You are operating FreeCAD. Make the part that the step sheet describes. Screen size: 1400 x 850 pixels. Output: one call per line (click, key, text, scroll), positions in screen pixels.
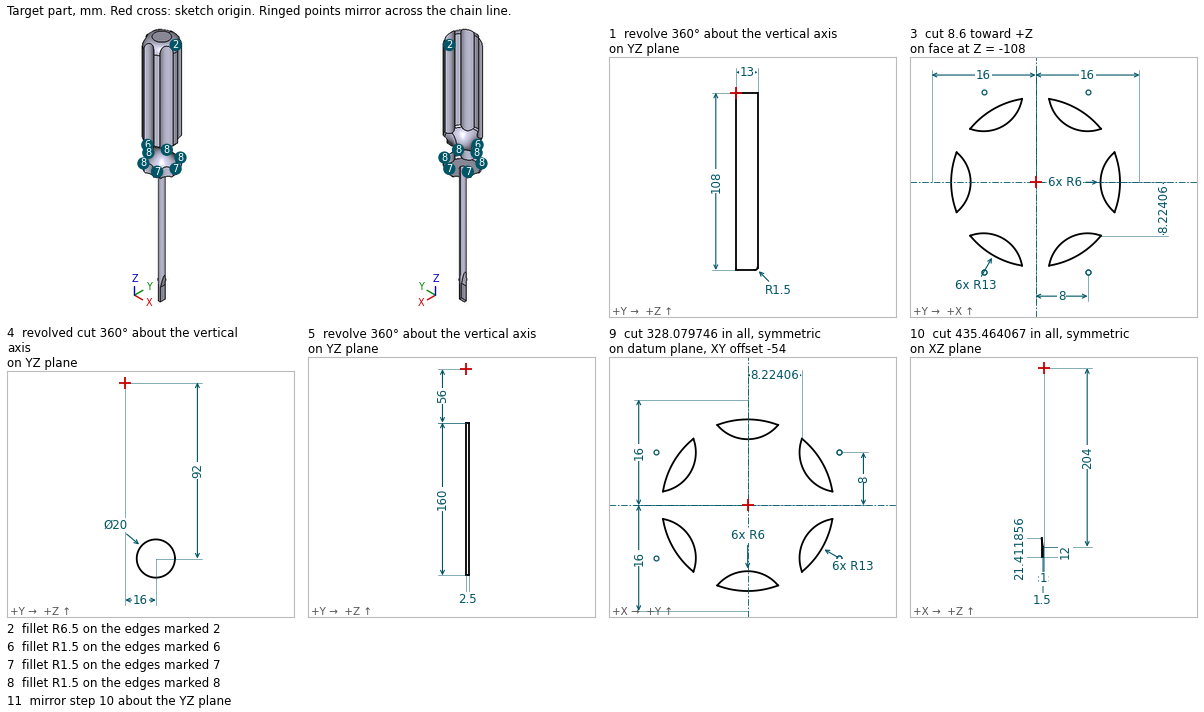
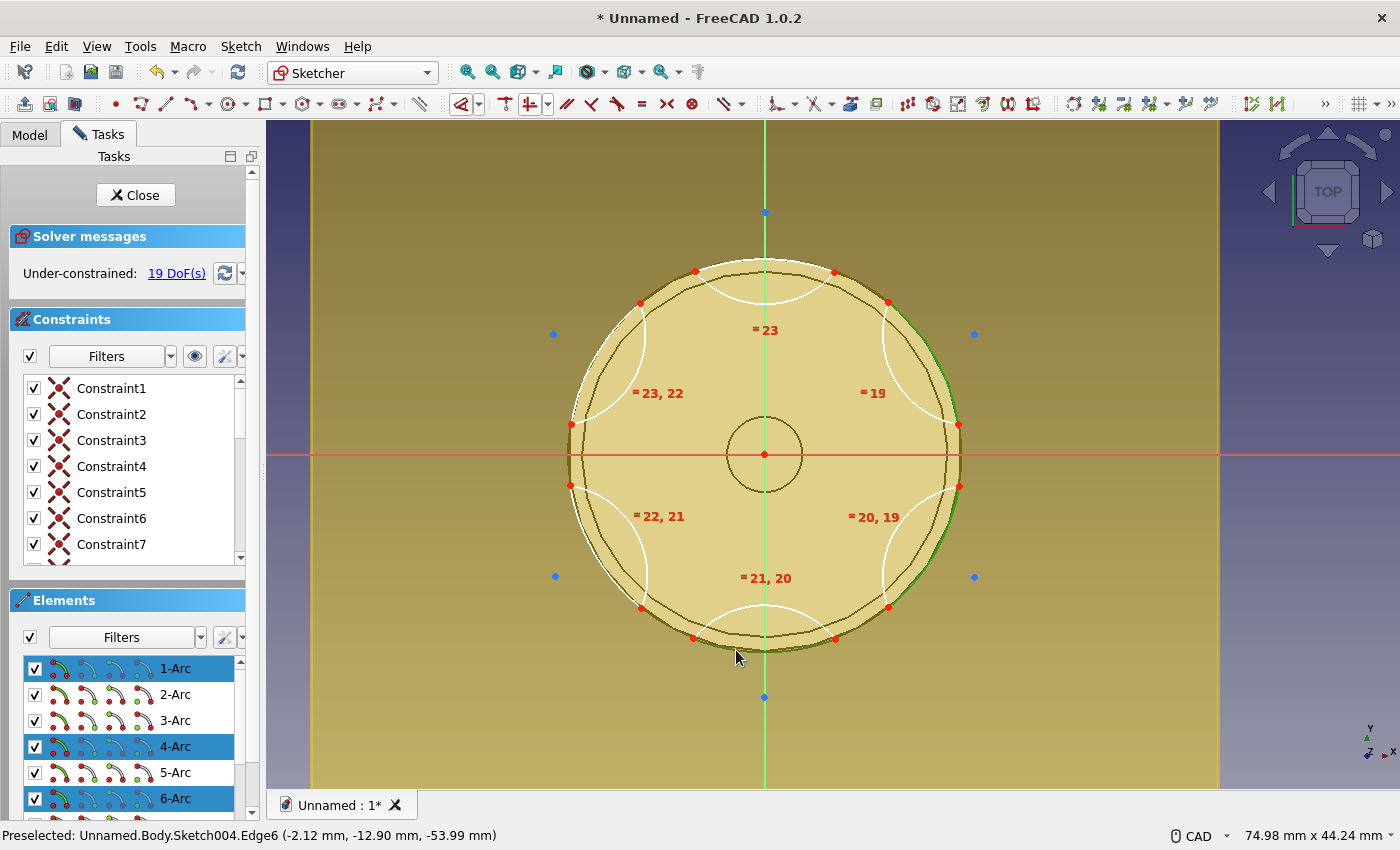
click(582, 528)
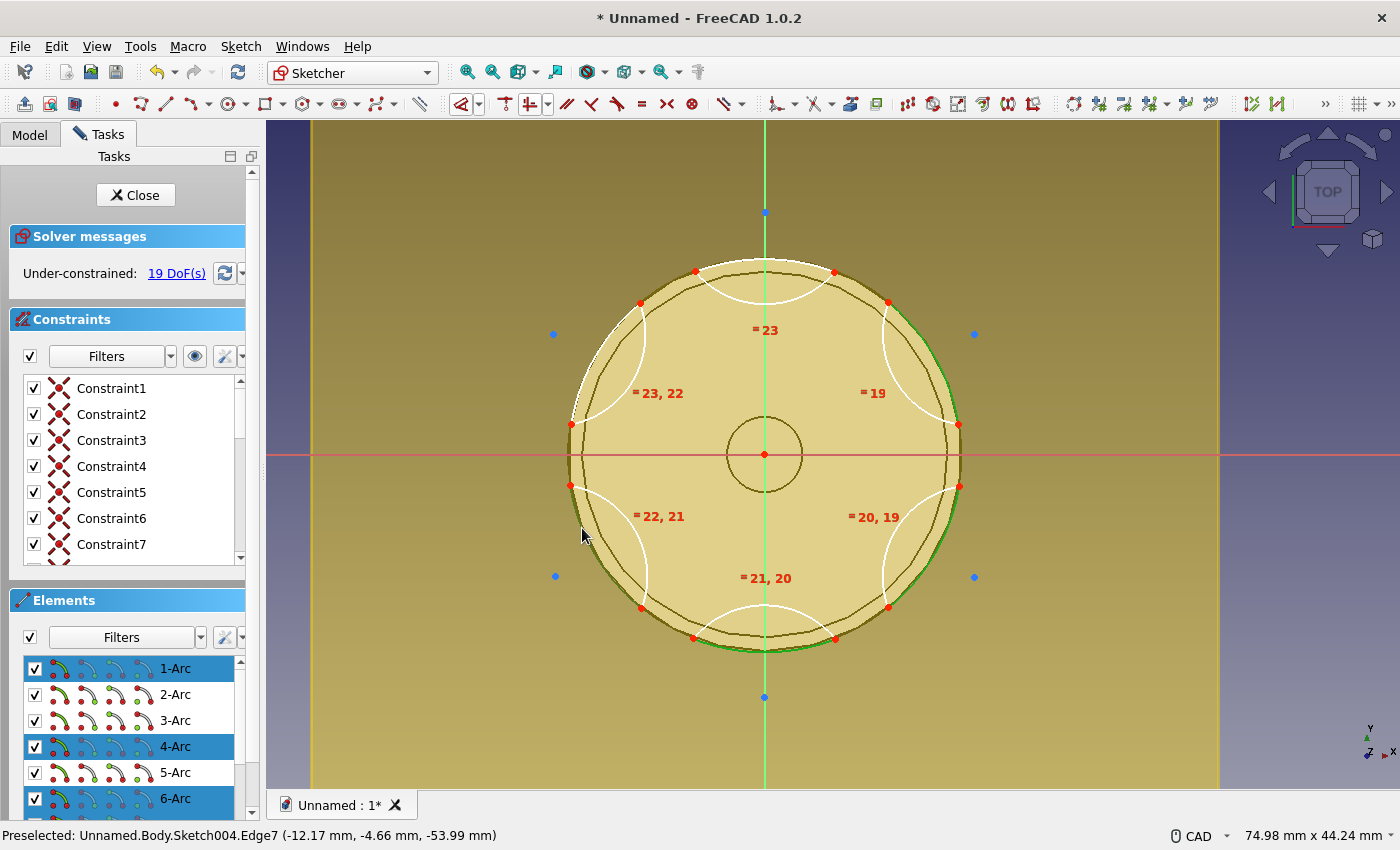
click(610, 334)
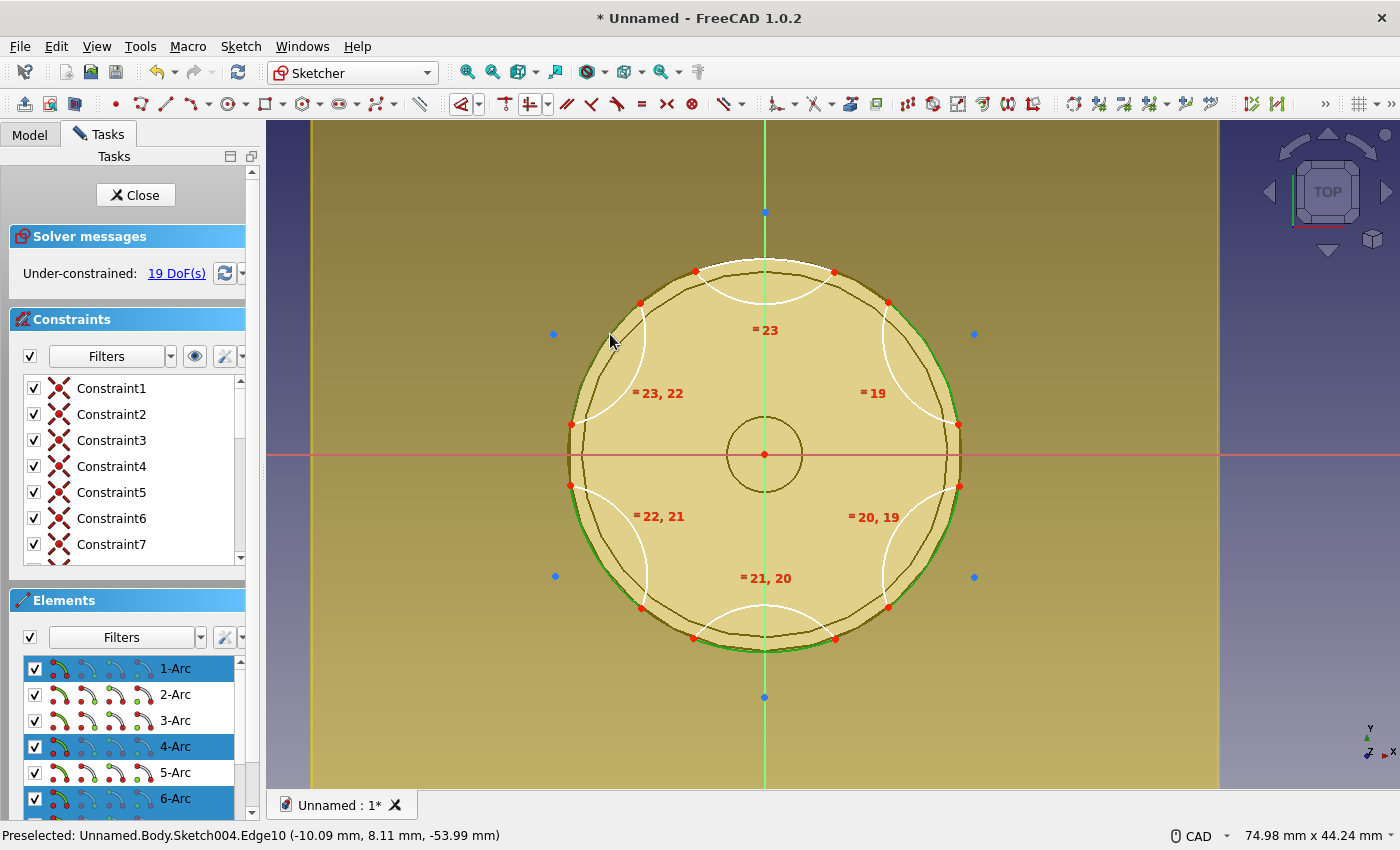
click(793, 261)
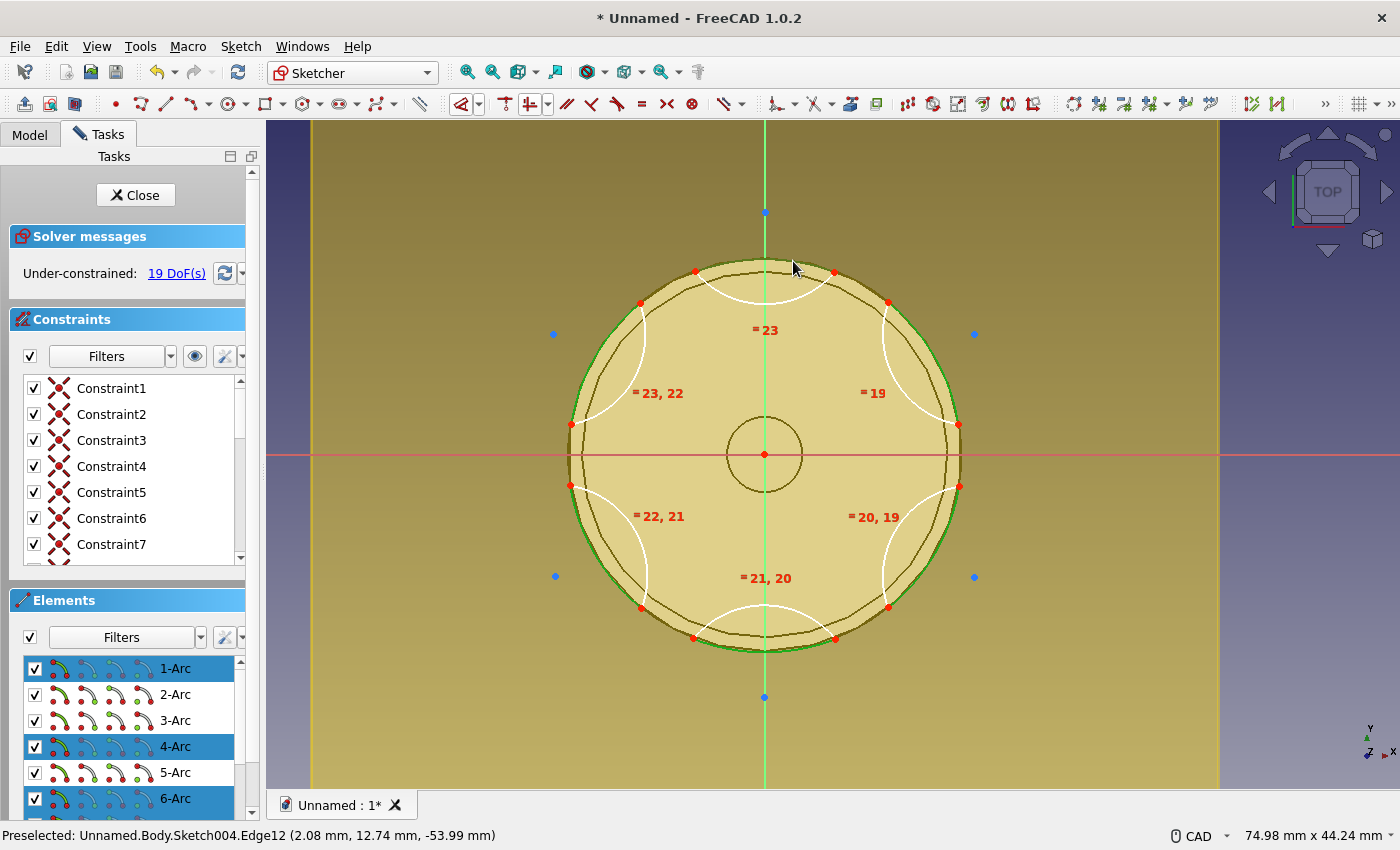
click(642, 104)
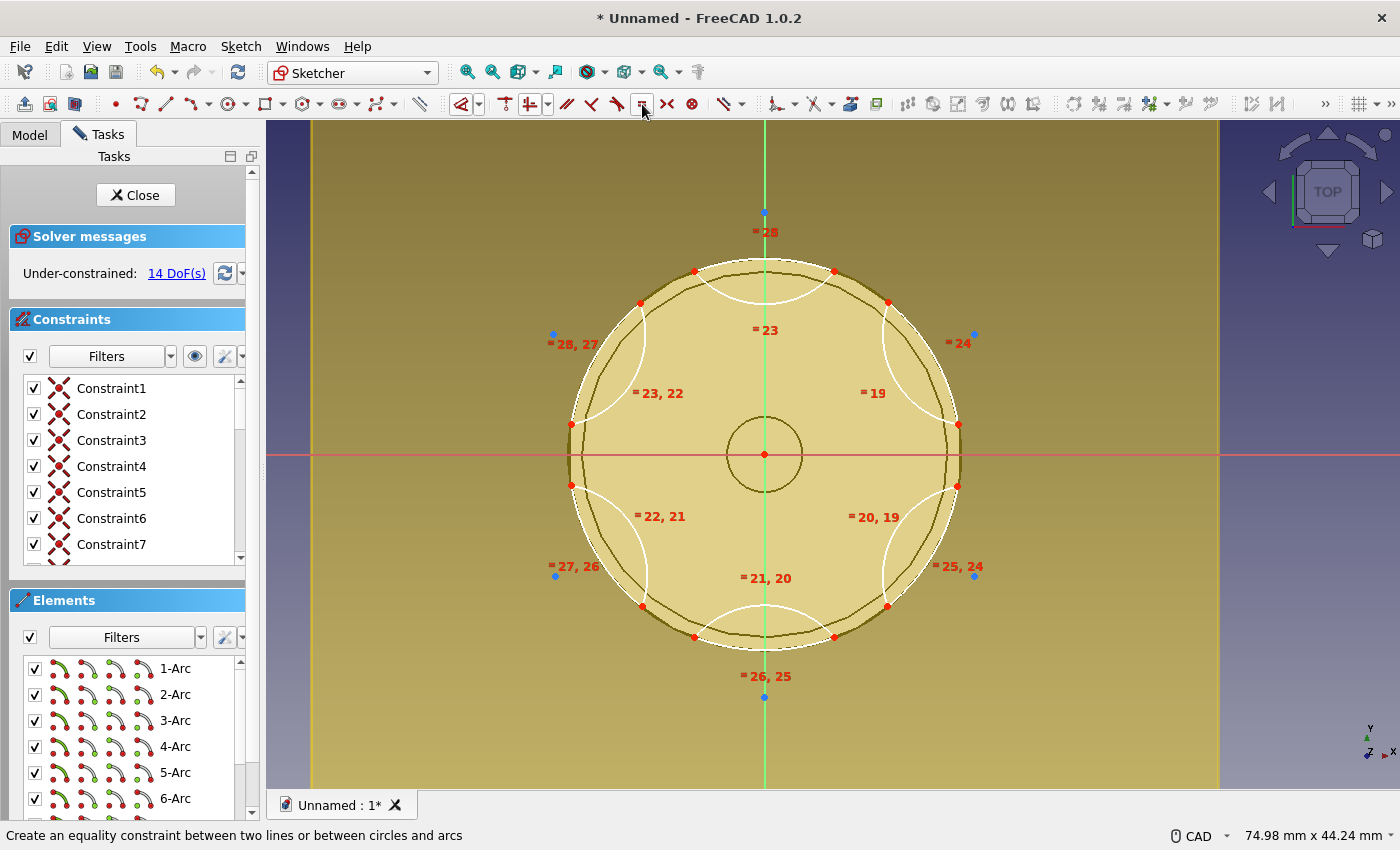
click(765, 697)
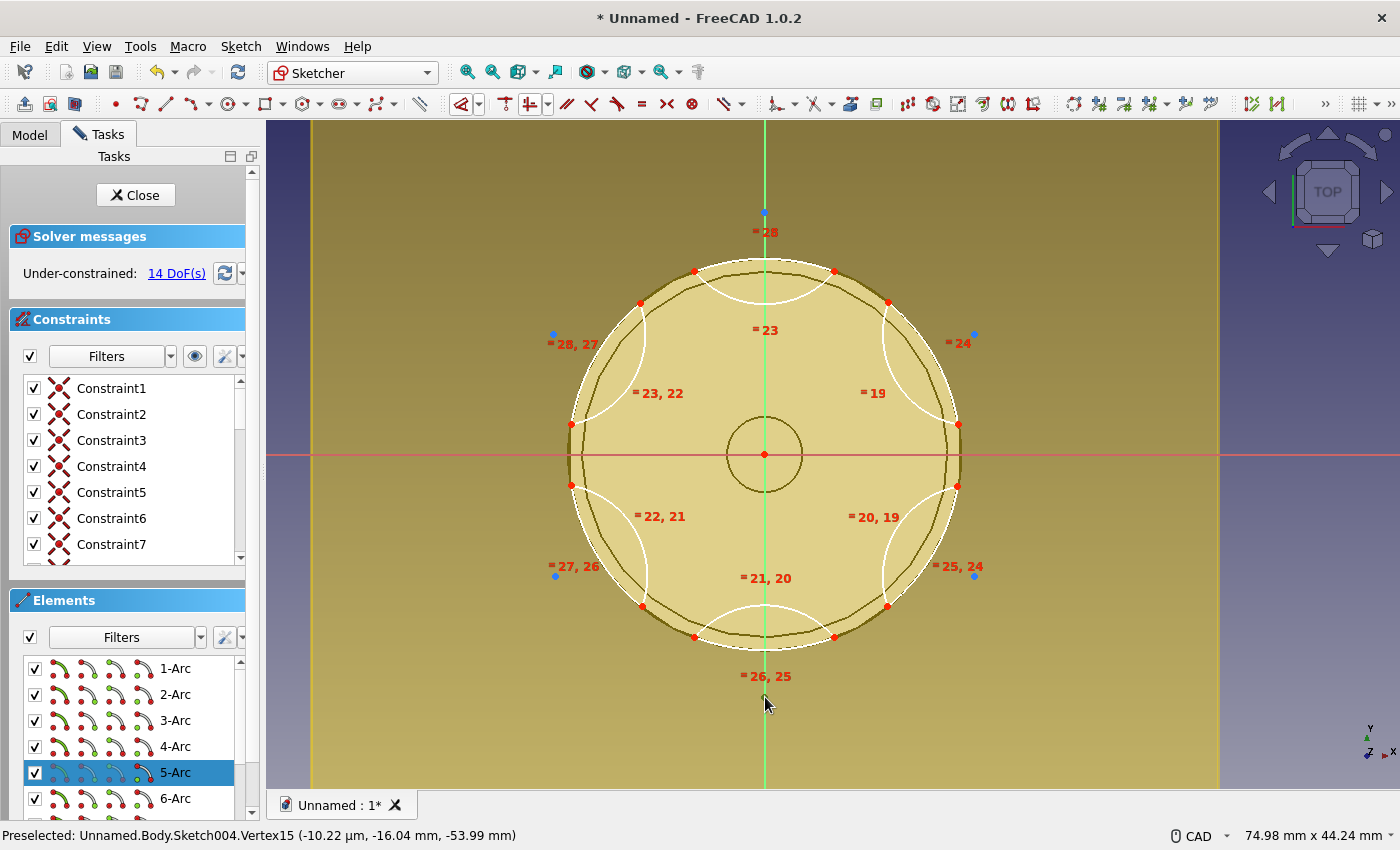
click(765, 717)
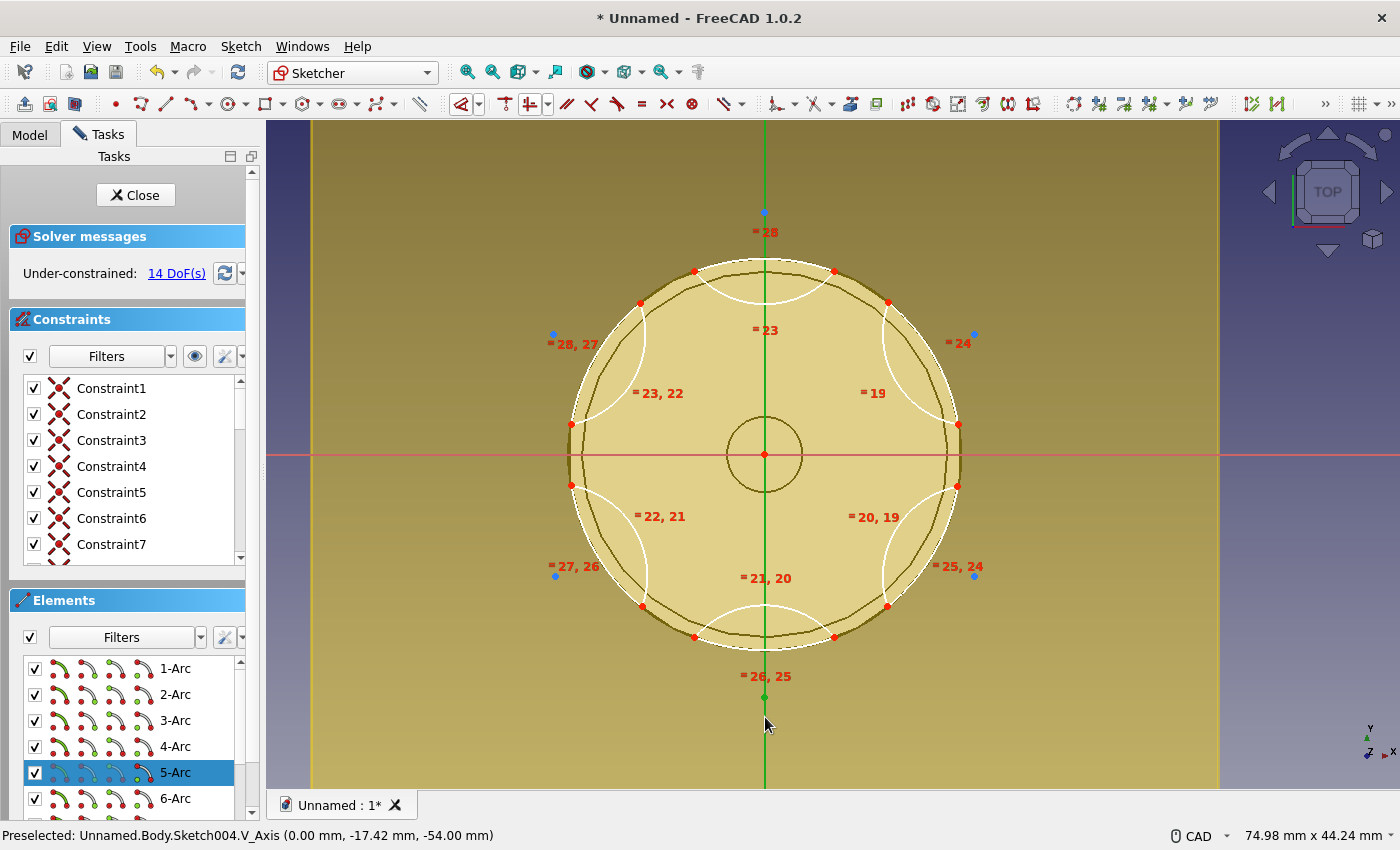
click(505, 104)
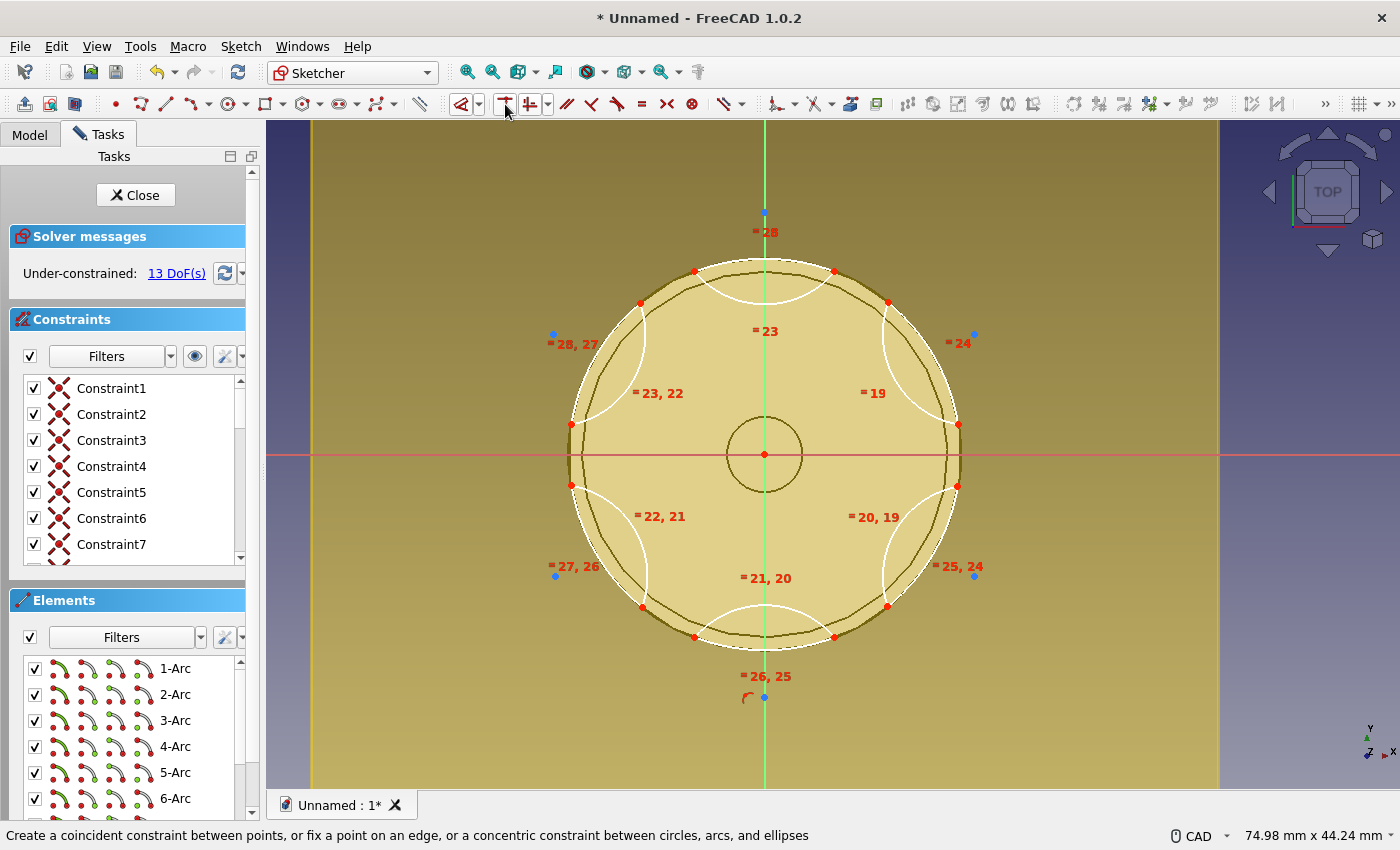
click(765, 212)